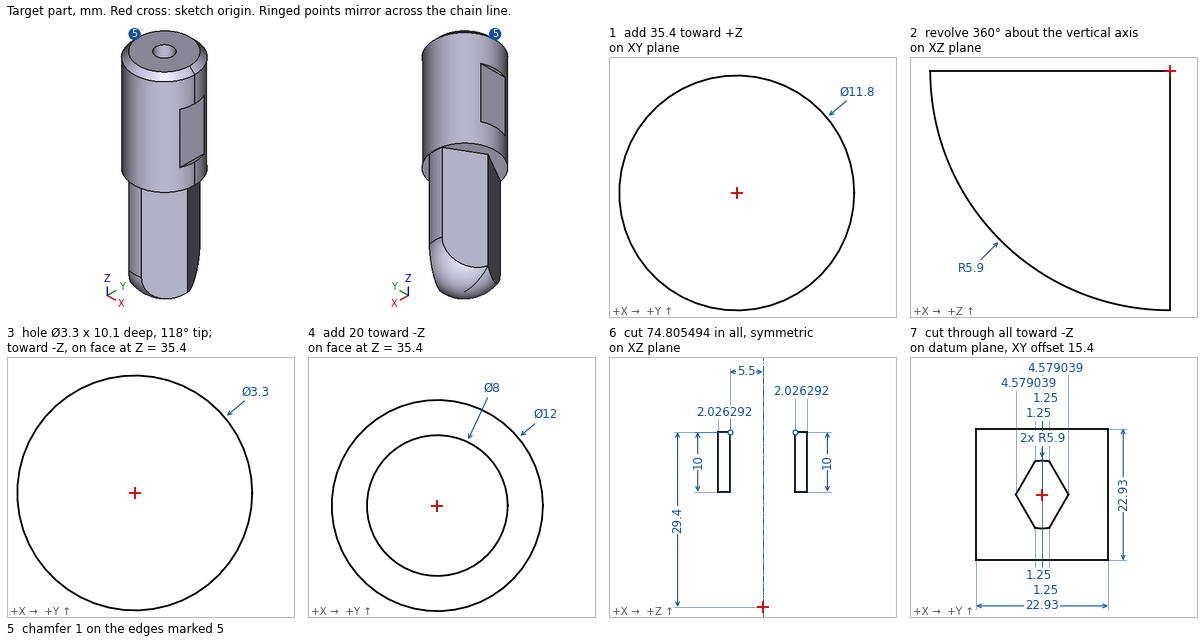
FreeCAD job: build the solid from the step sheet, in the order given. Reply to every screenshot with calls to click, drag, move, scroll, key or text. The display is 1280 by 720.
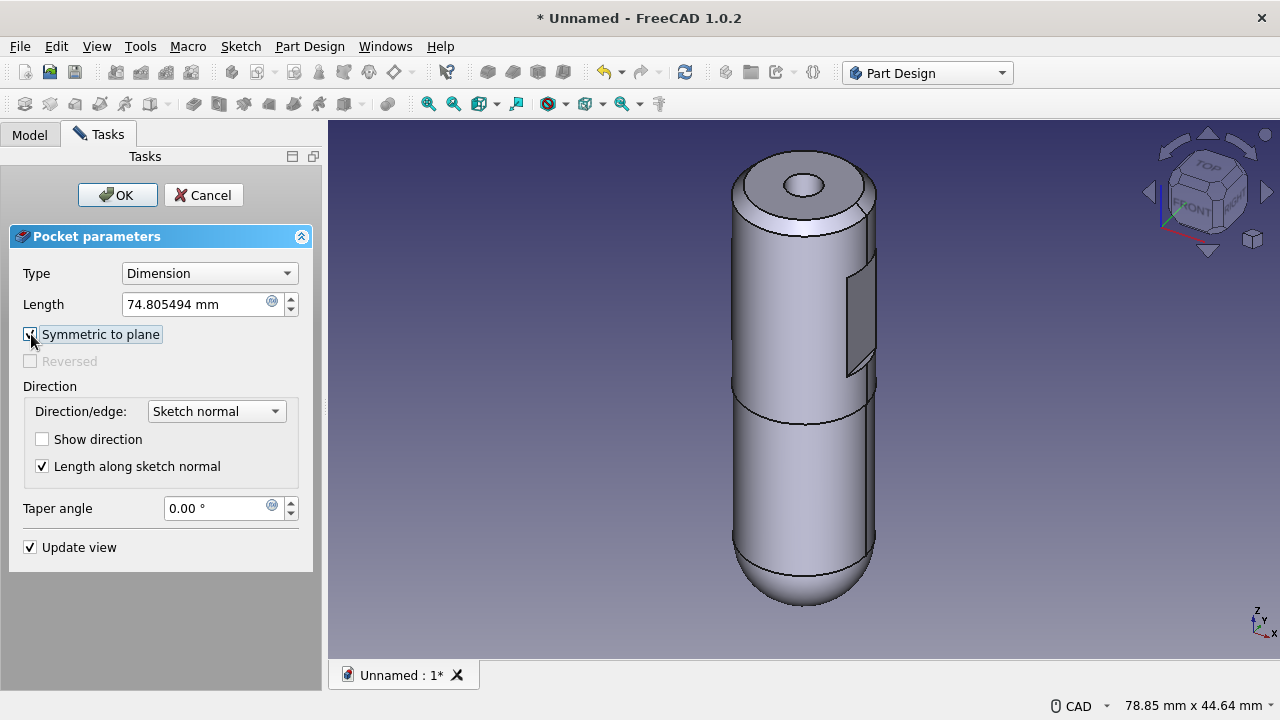
click(118, 195)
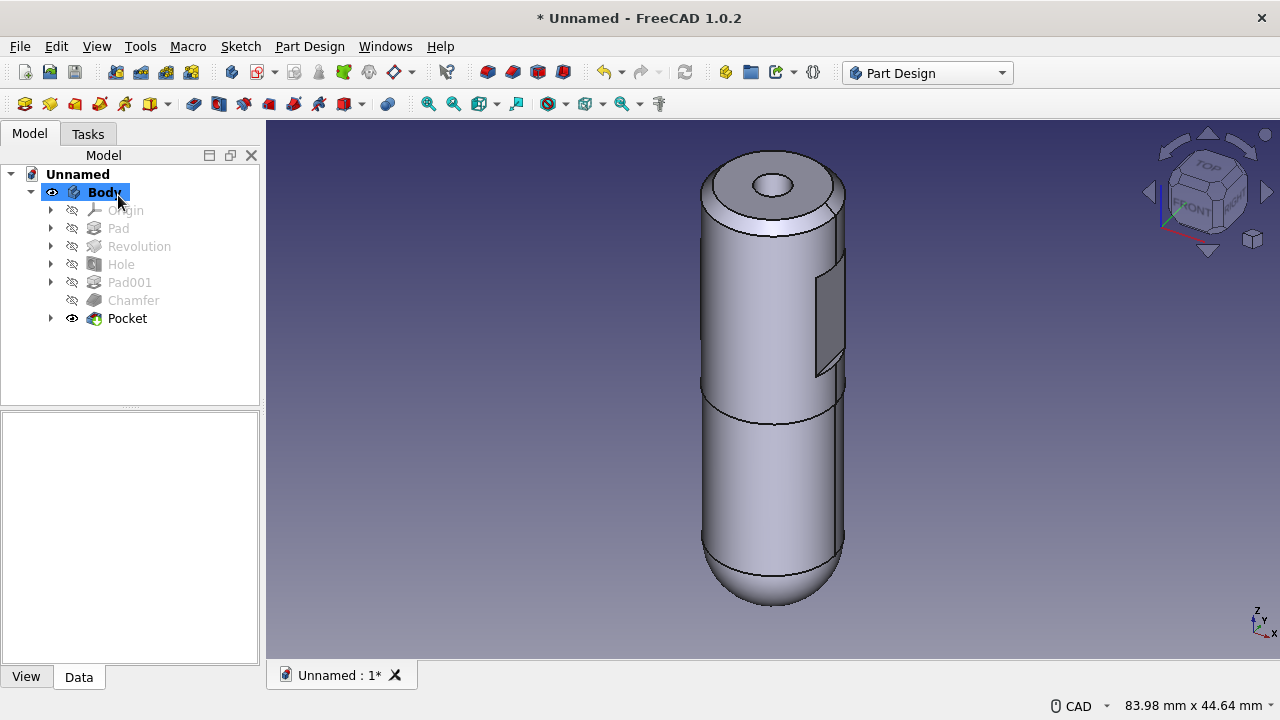
key(5)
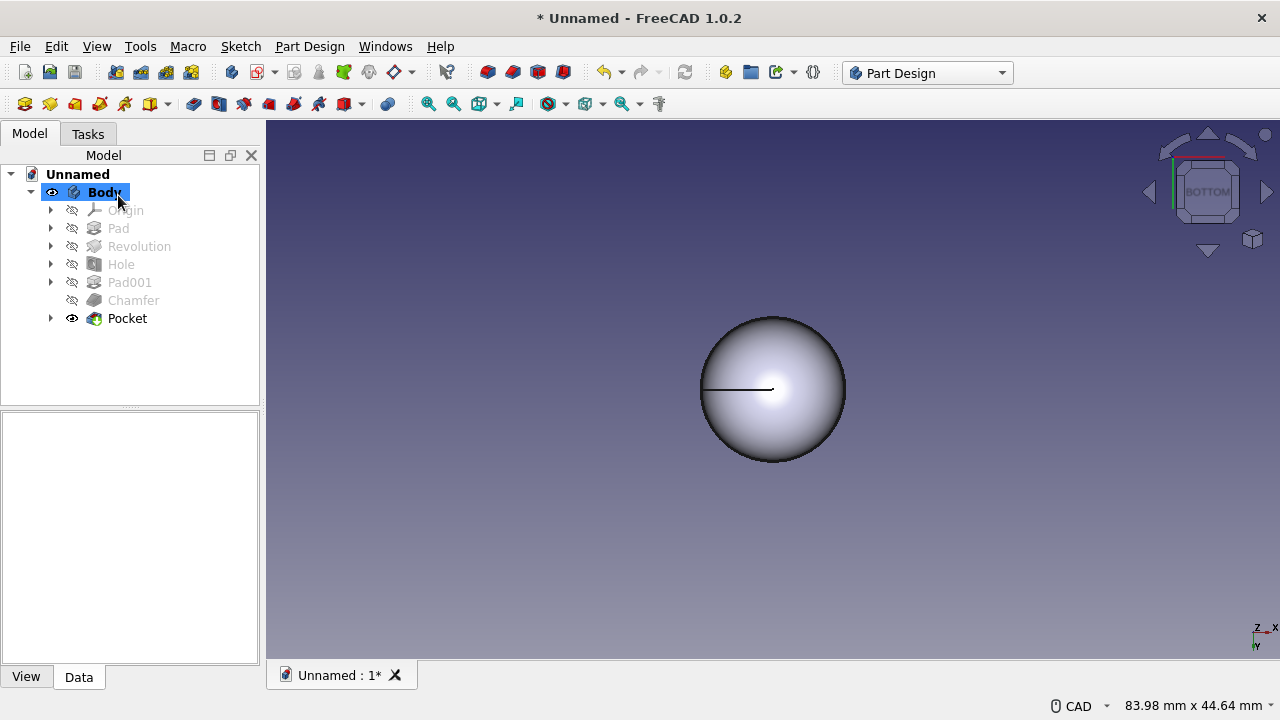
key(v)
key(f)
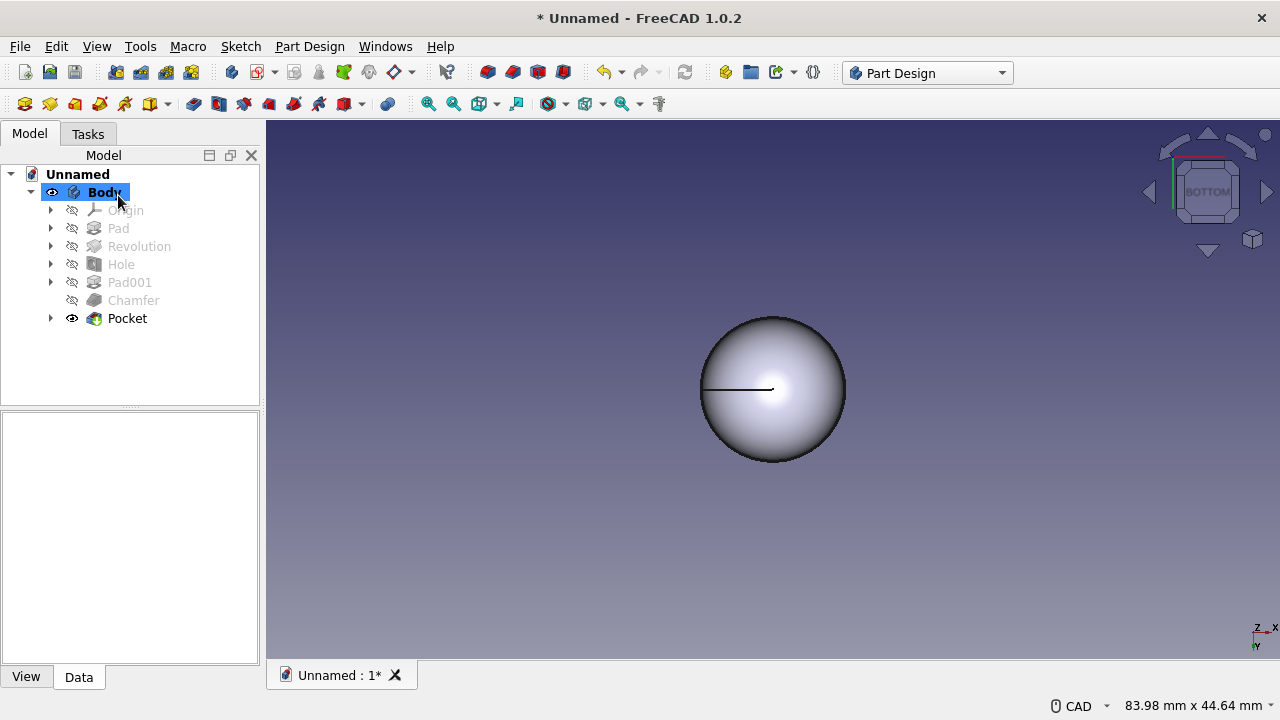
scroll(837, 355, up, 15)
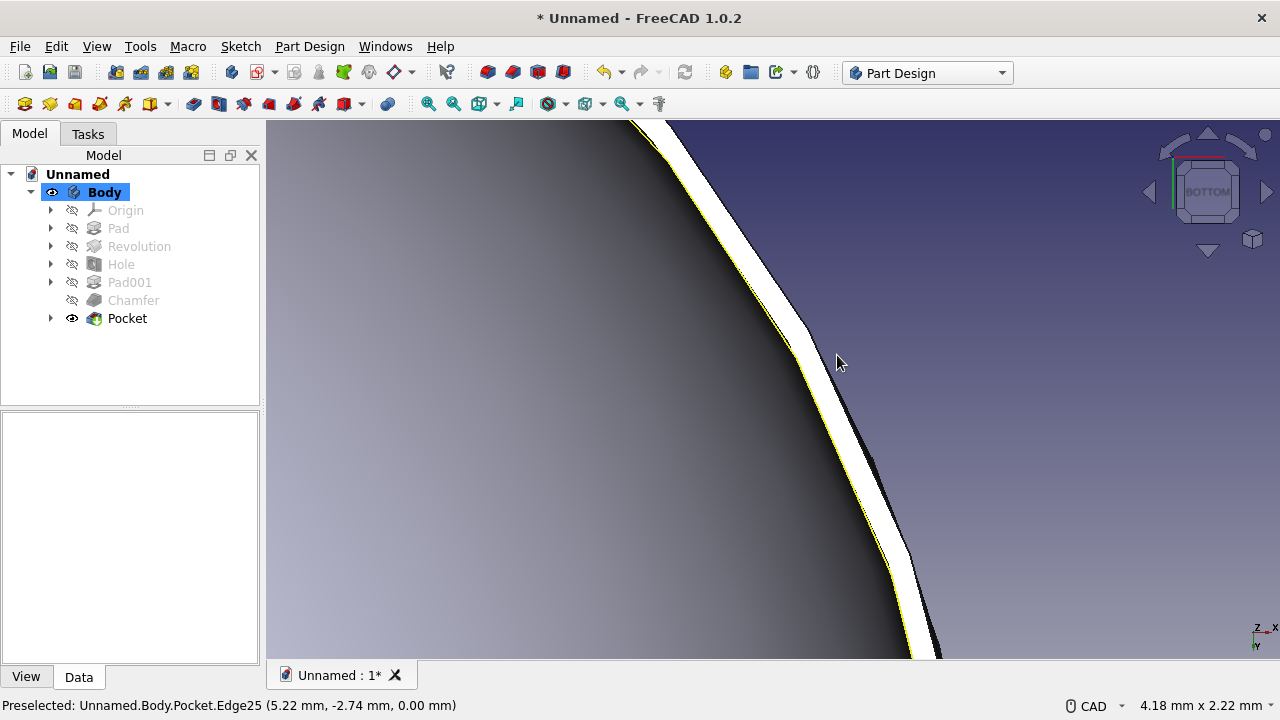
click(429, 104)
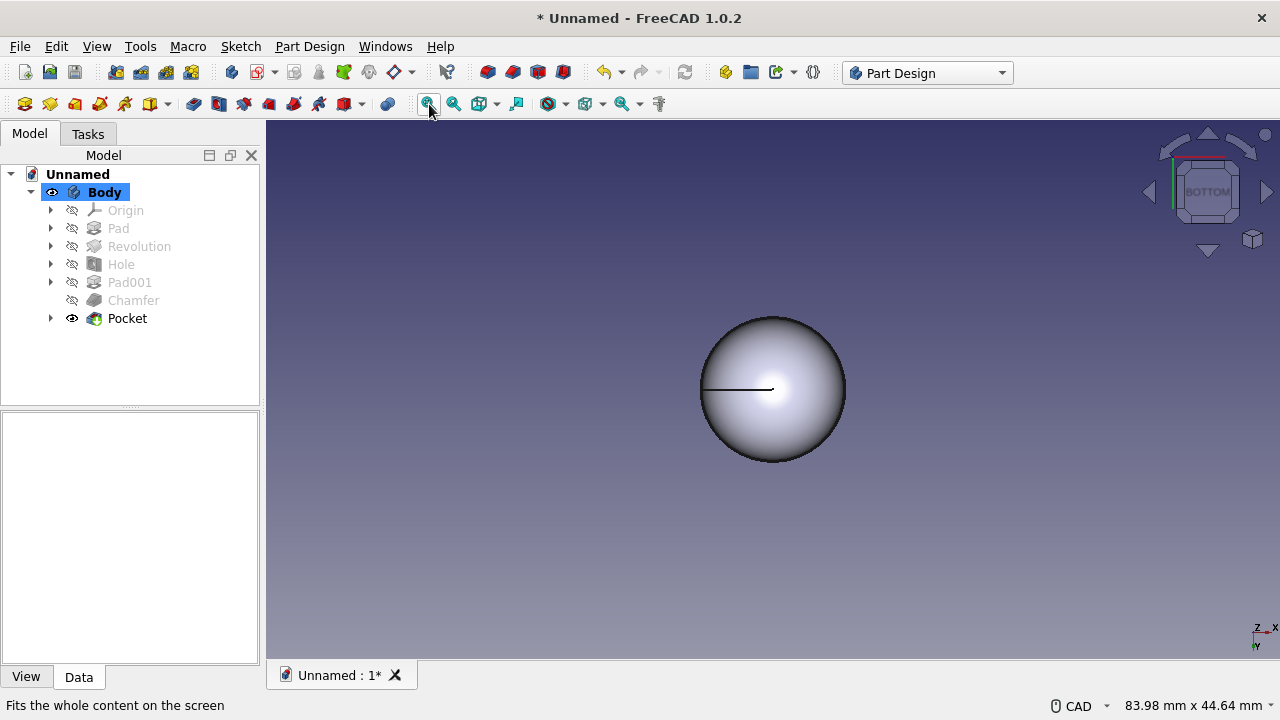
key(1)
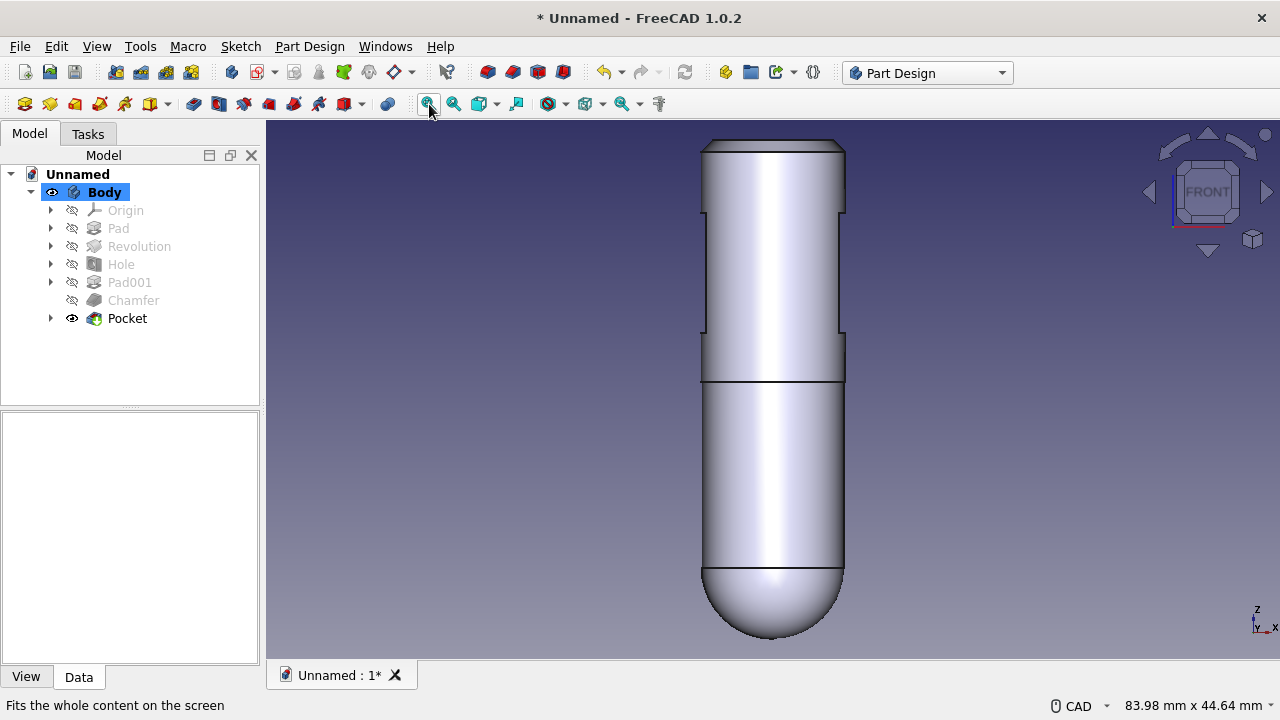
key(3)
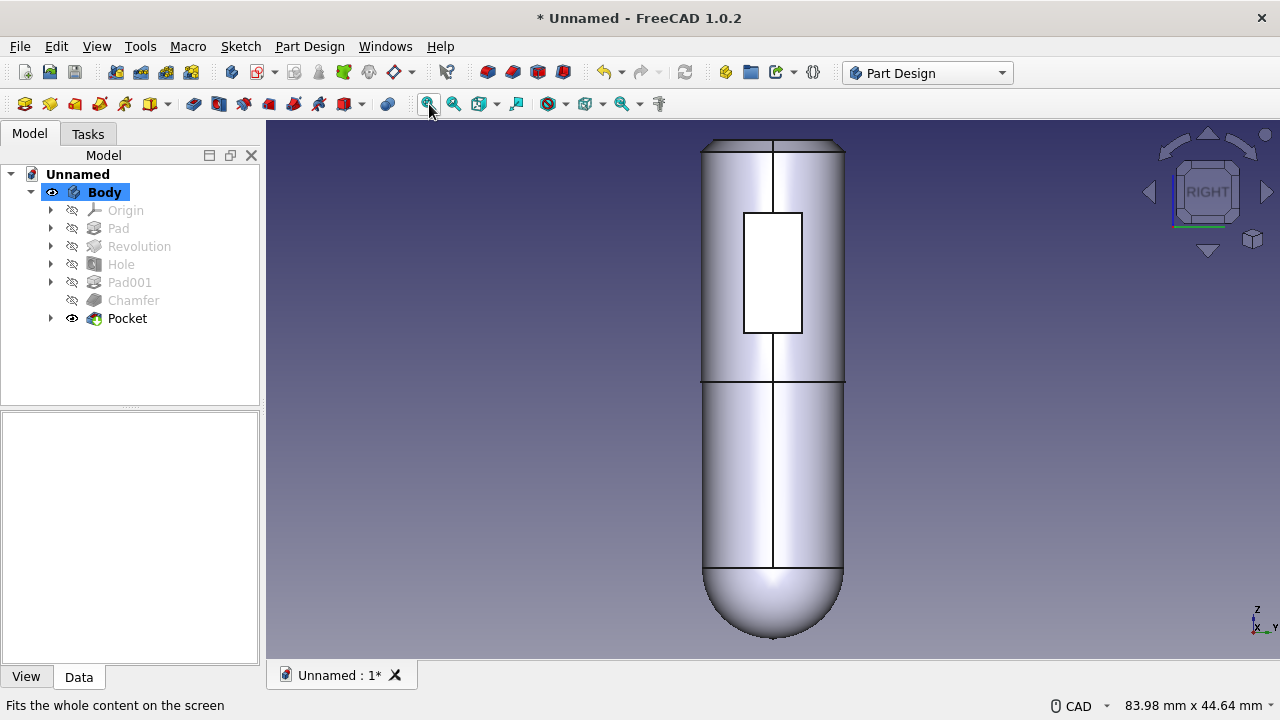
click(51, 210)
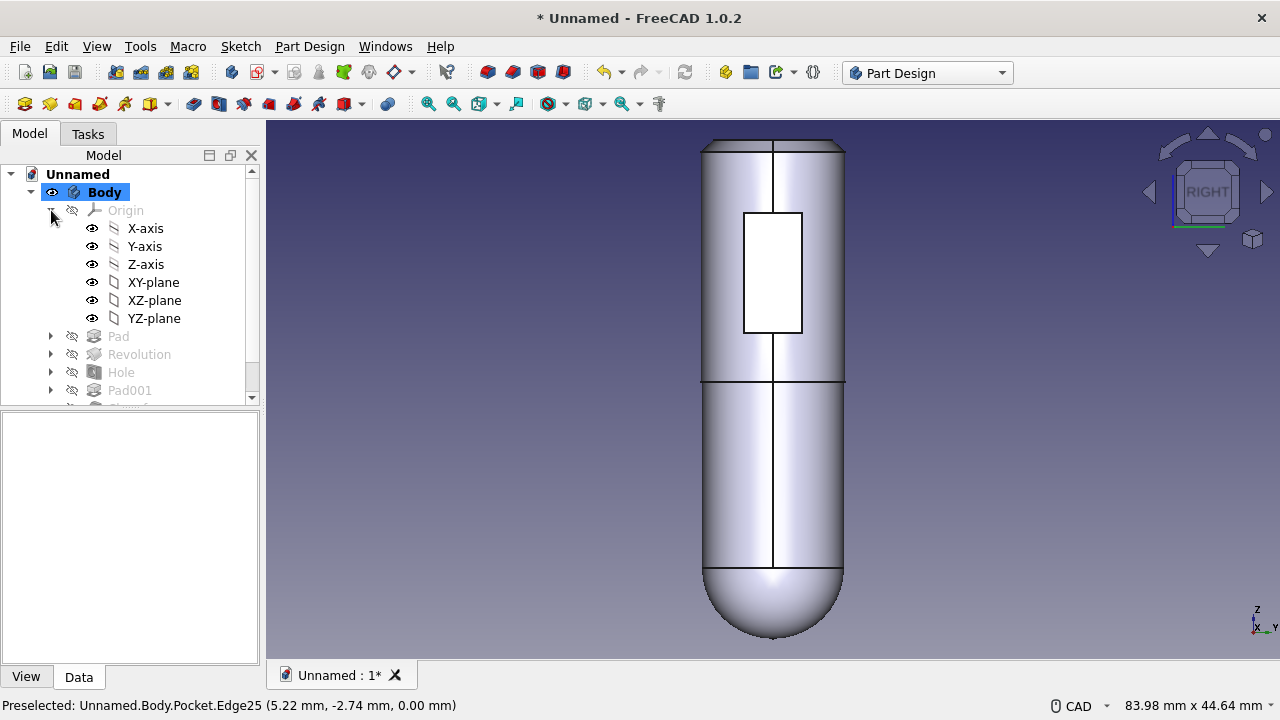
click(137, 282)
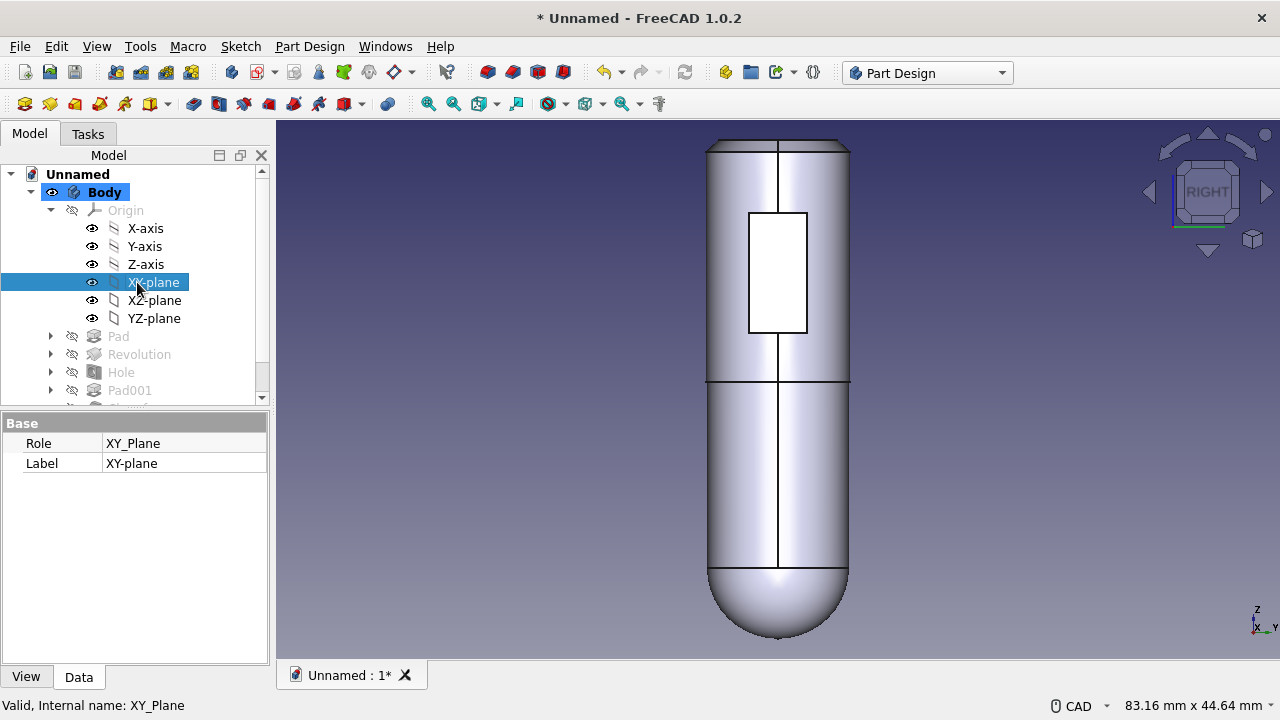
click(394, 72)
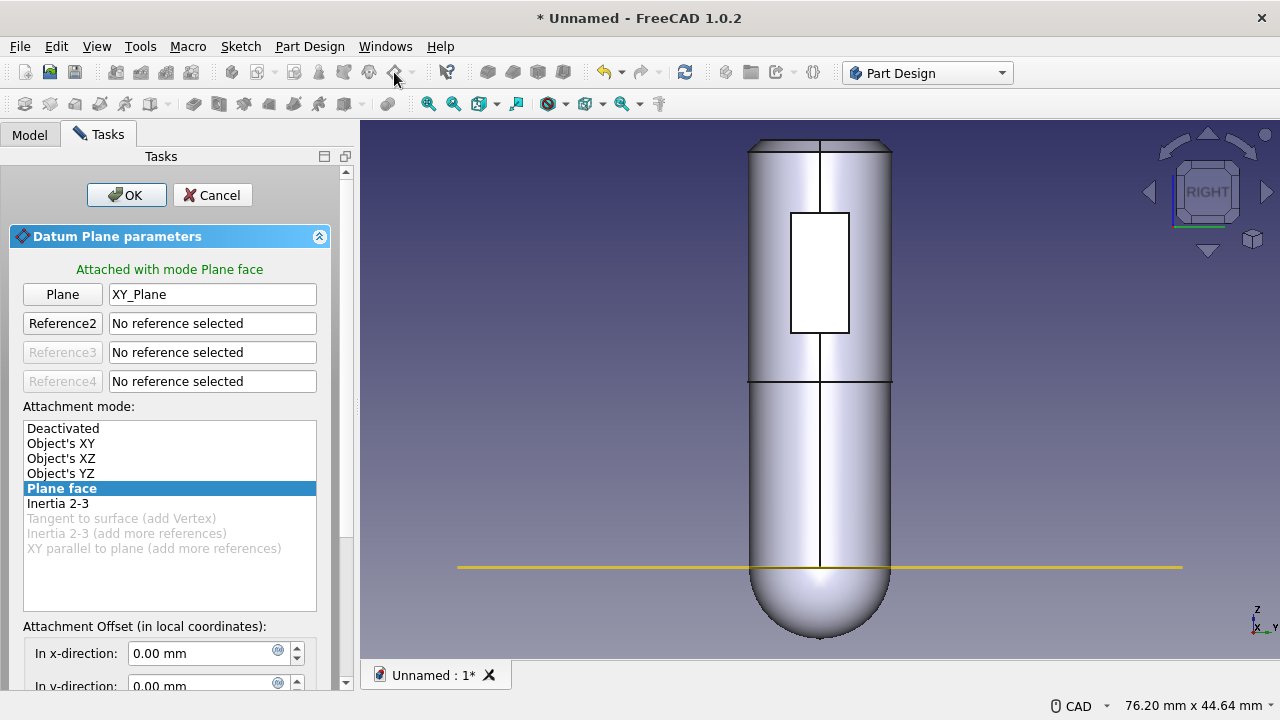
scroll(346, 428, down, 2)